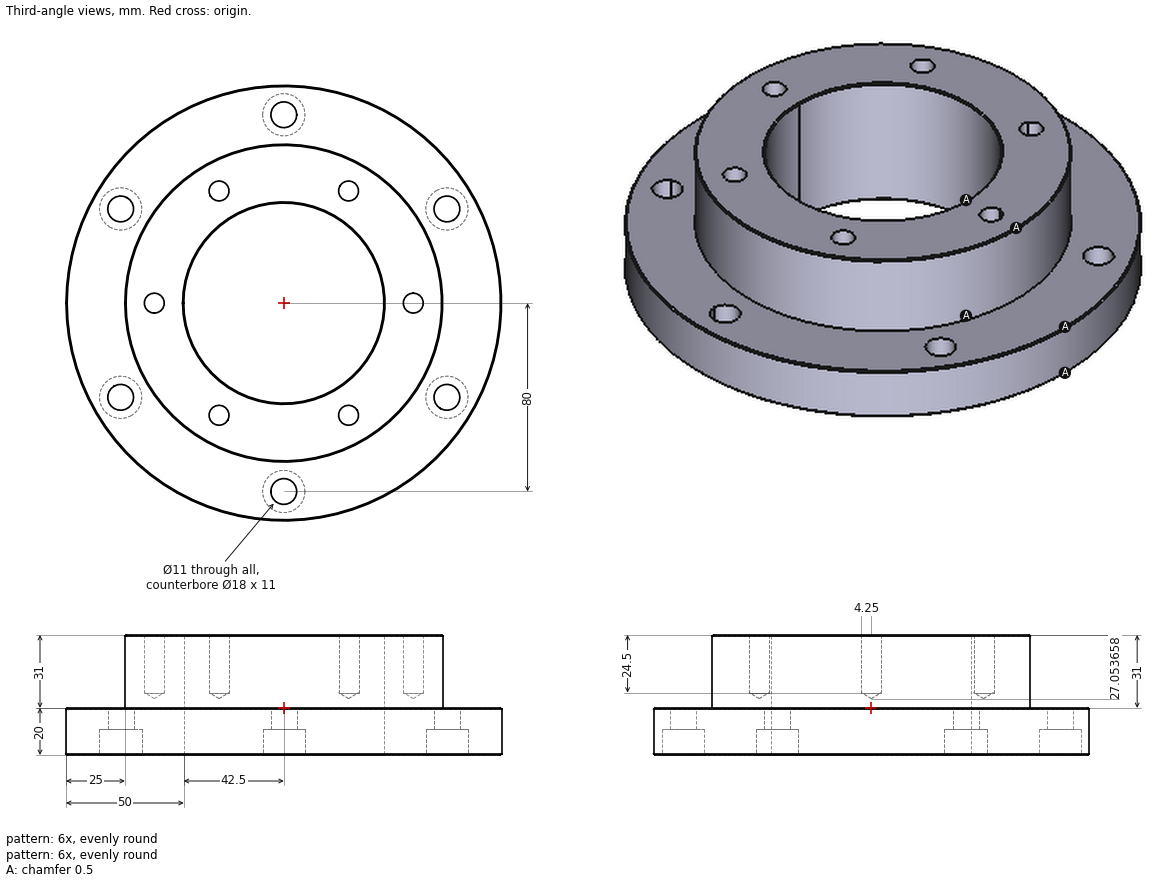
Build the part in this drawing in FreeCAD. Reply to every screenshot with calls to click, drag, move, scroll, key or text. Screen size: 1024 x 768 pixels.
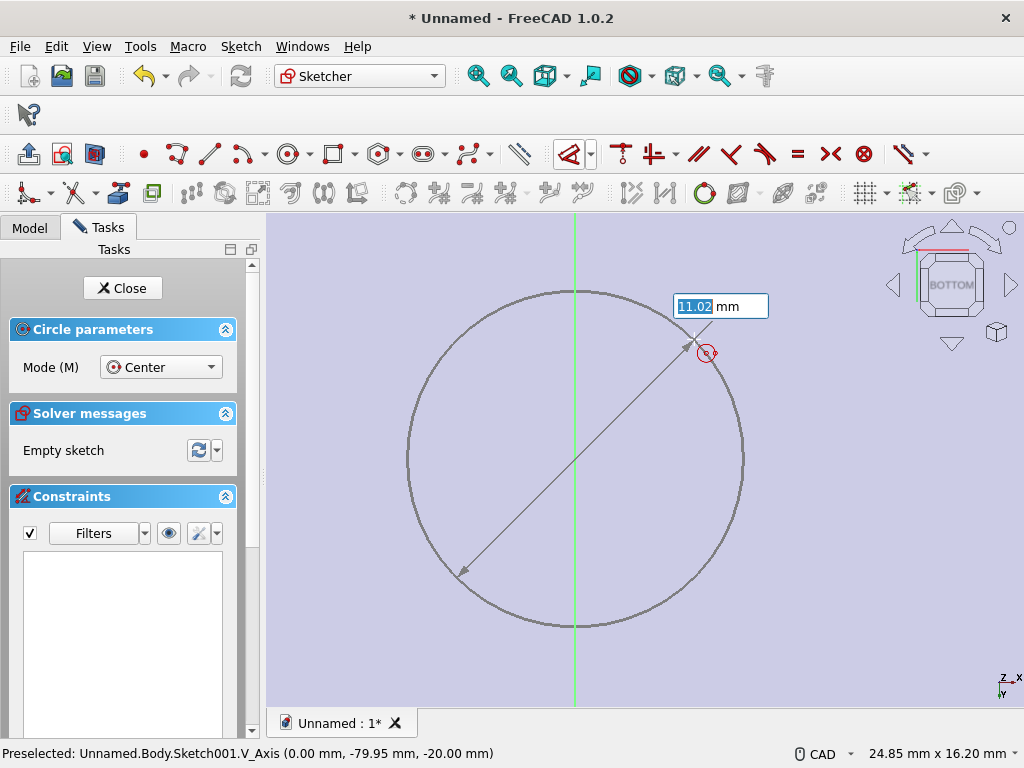
text(11)
key(Return)
key(Escape)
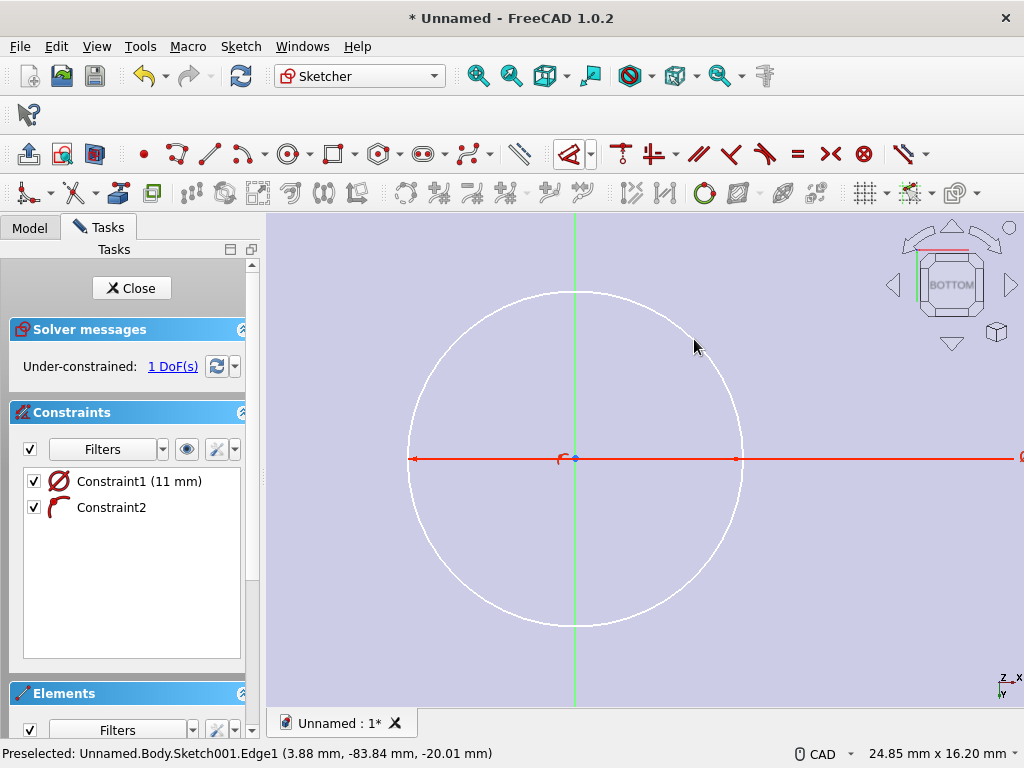
click(575, 459)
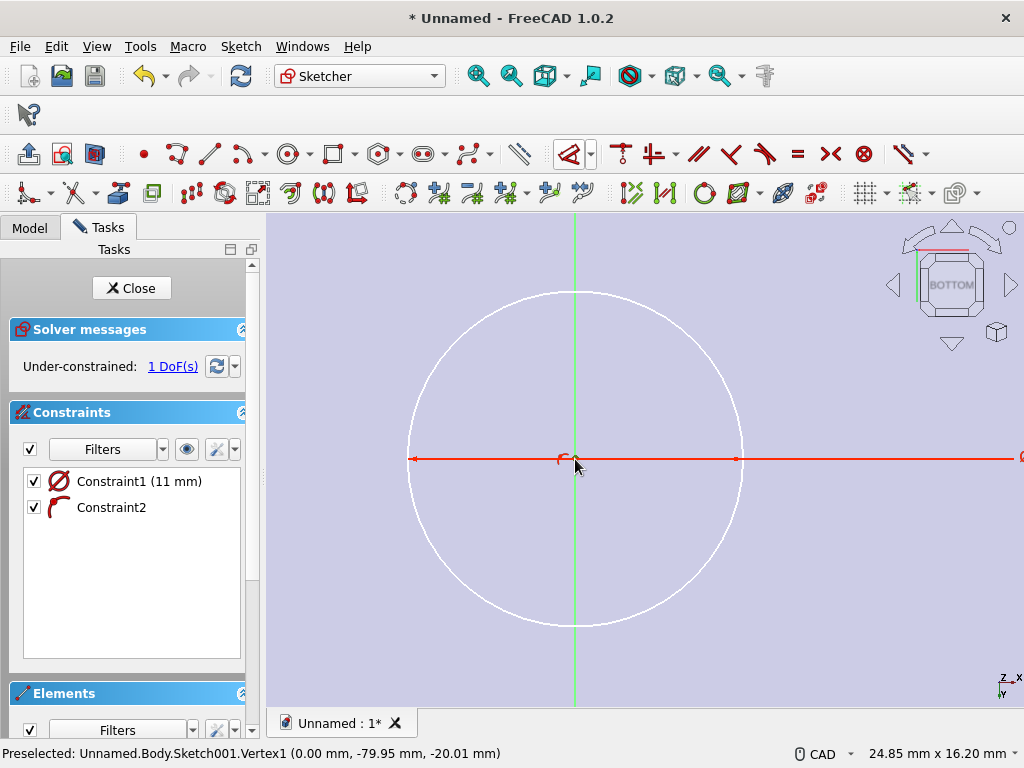
key(i)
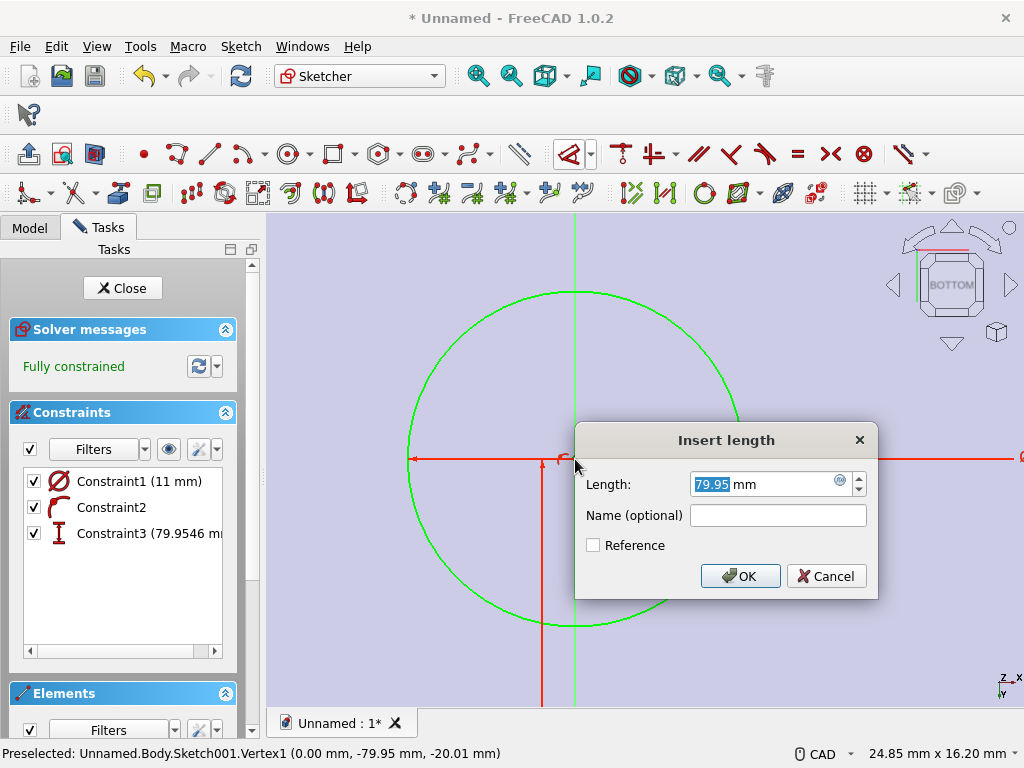
text(80)
key(Return)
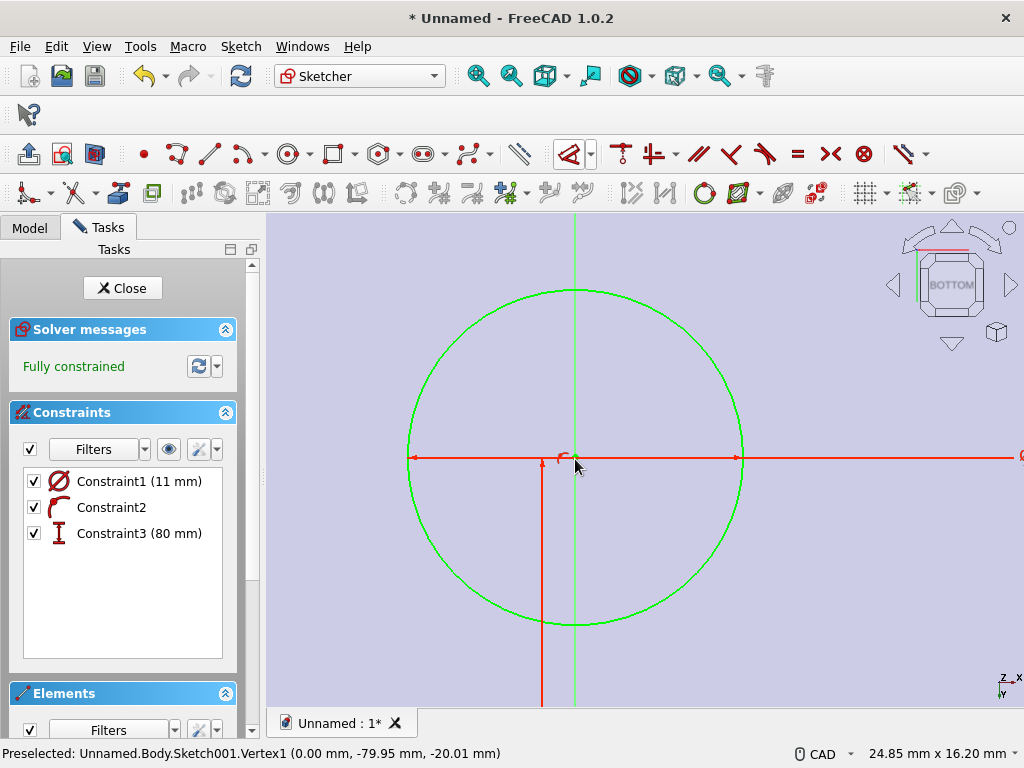
click(123, 288)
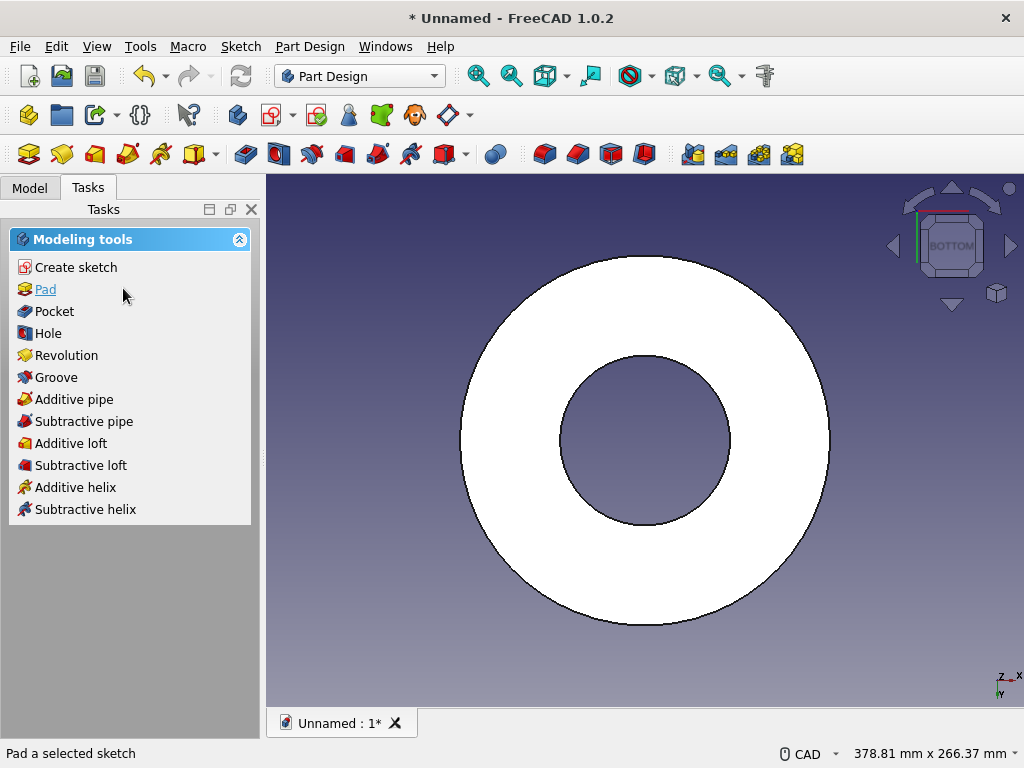
click(279, 154)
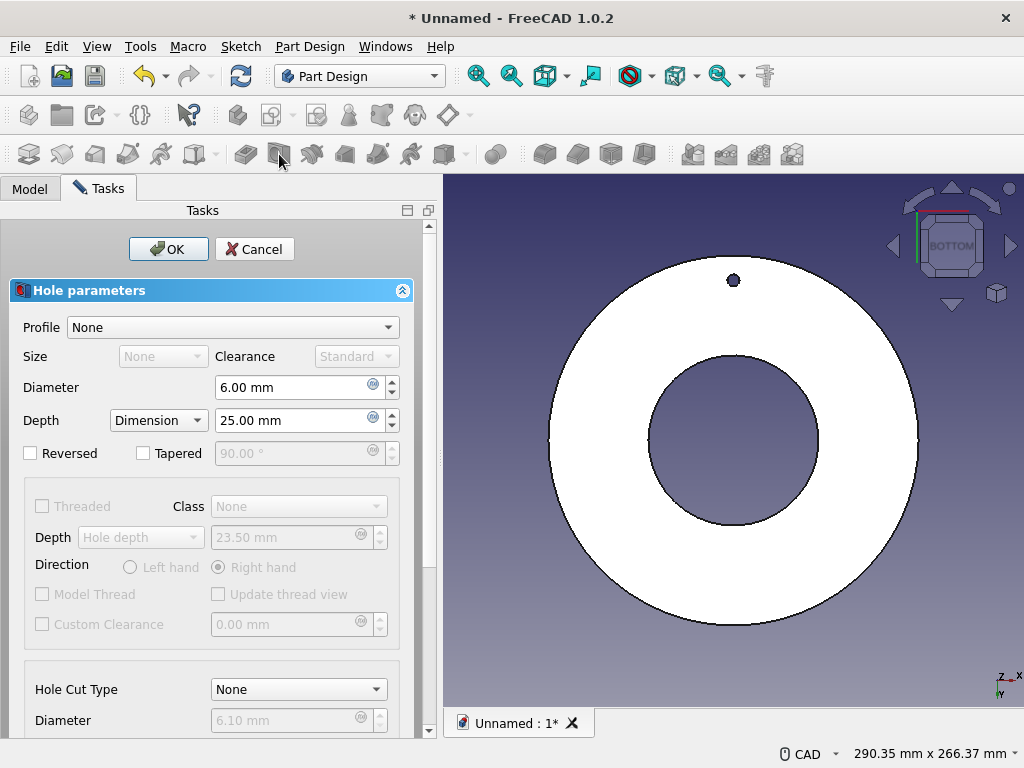
triple_click(300, 388)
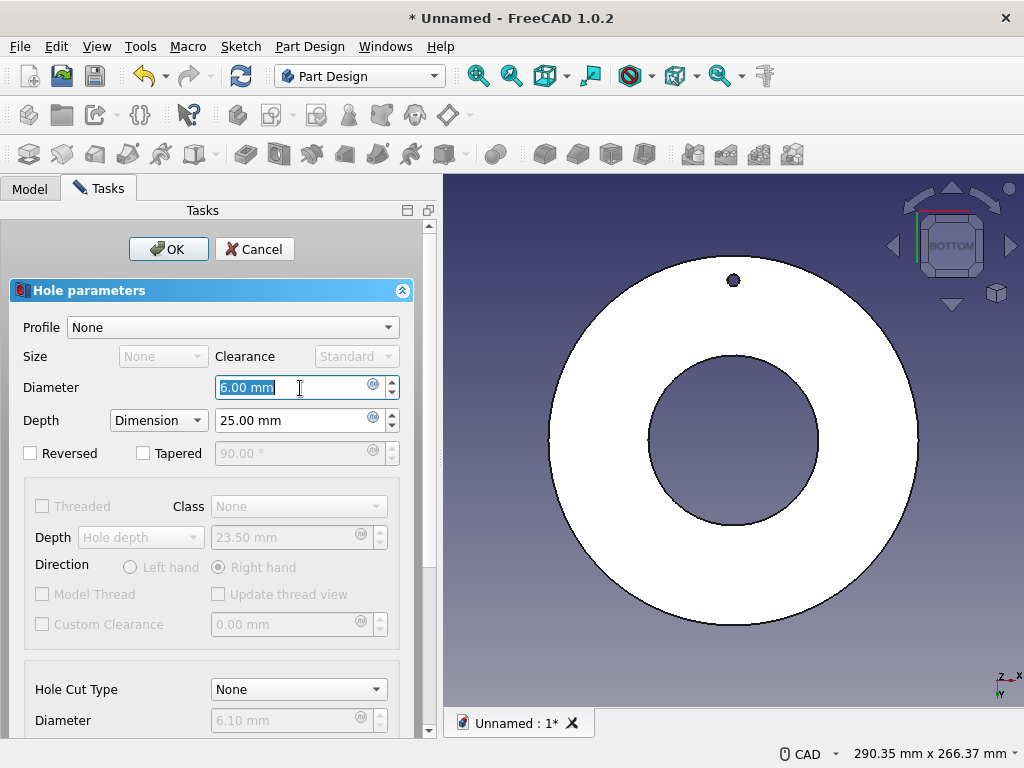
text(11)
key(Tab)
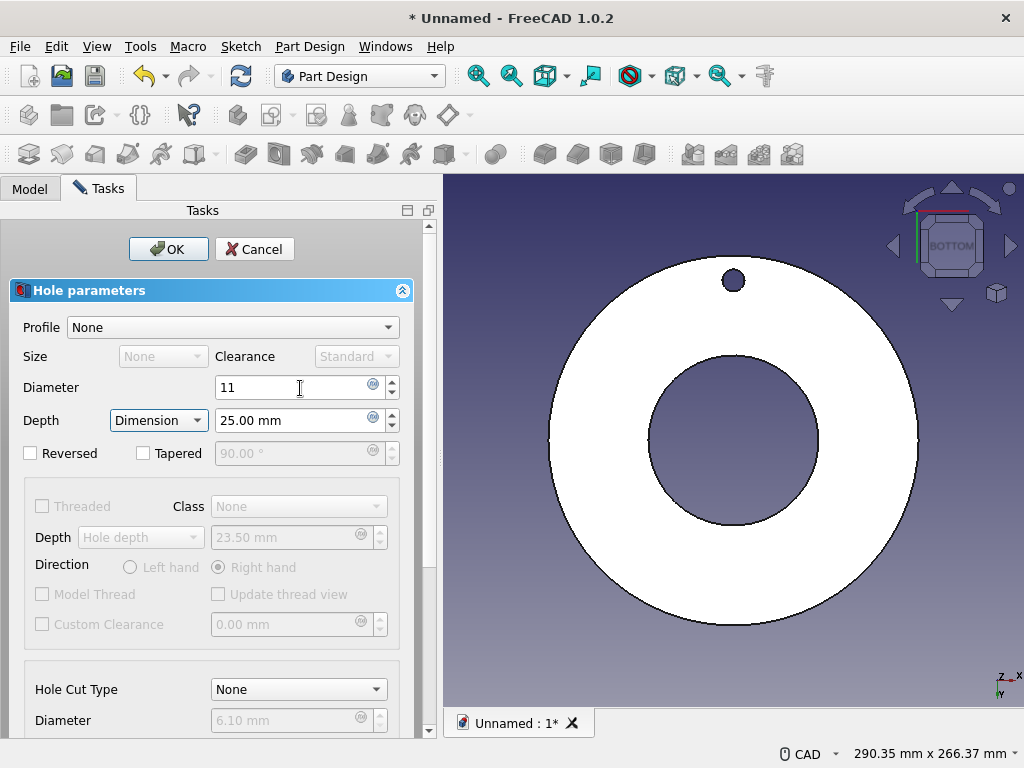
click(160, 420)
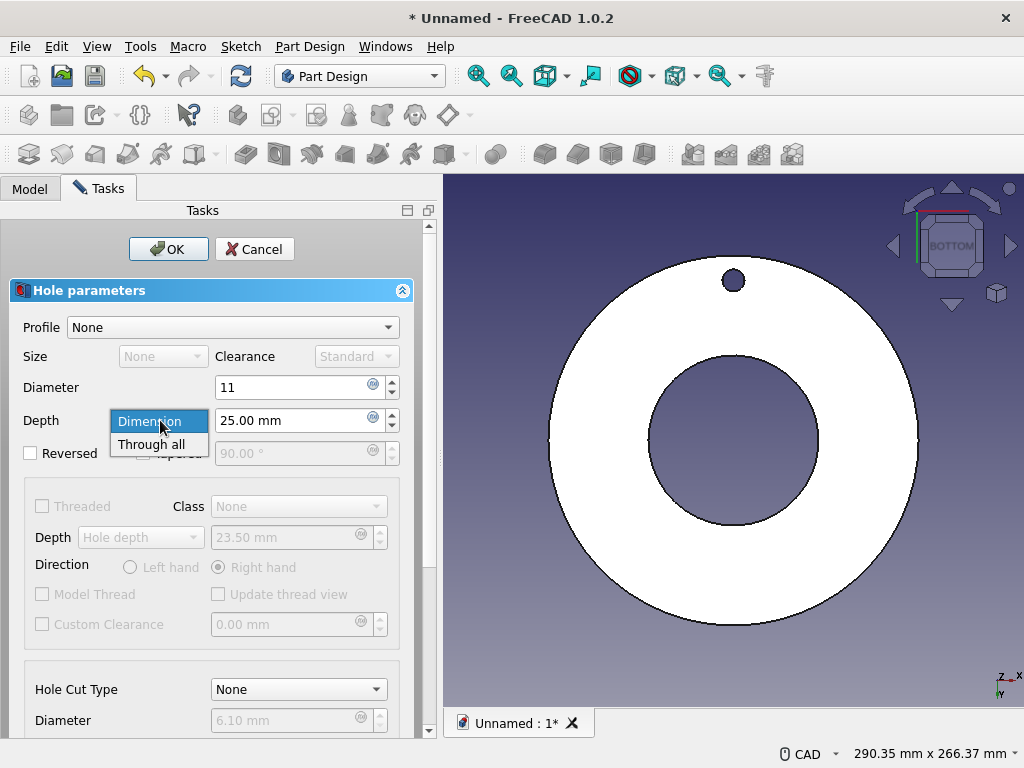
click(158, 444)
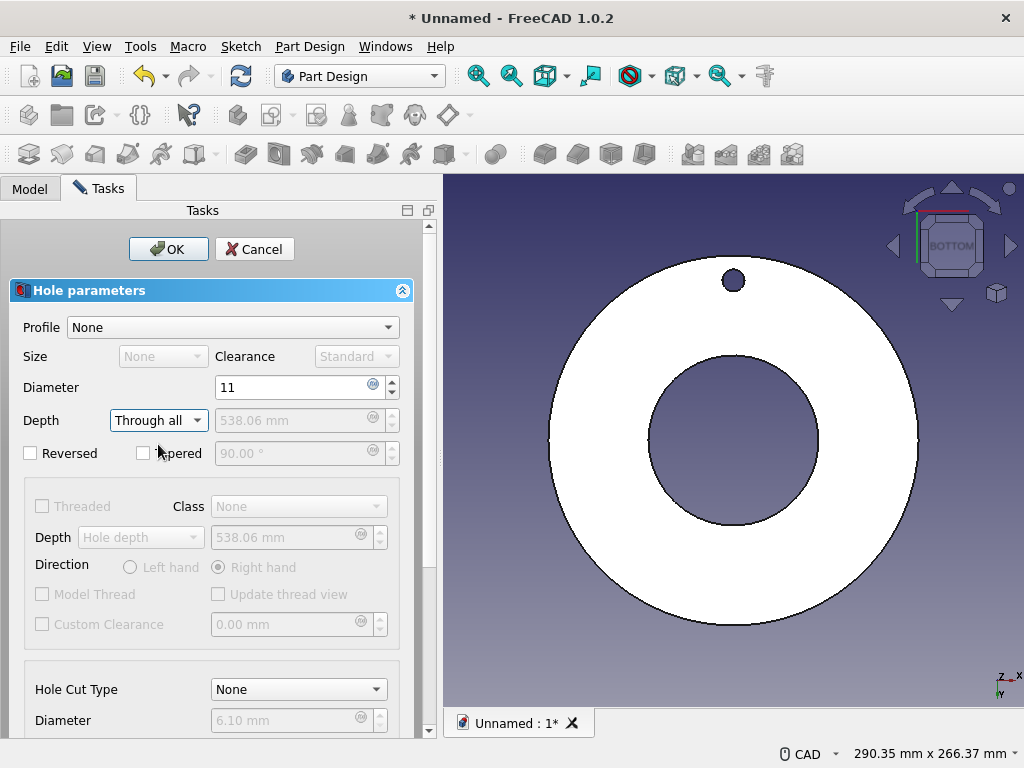
click(300, 690)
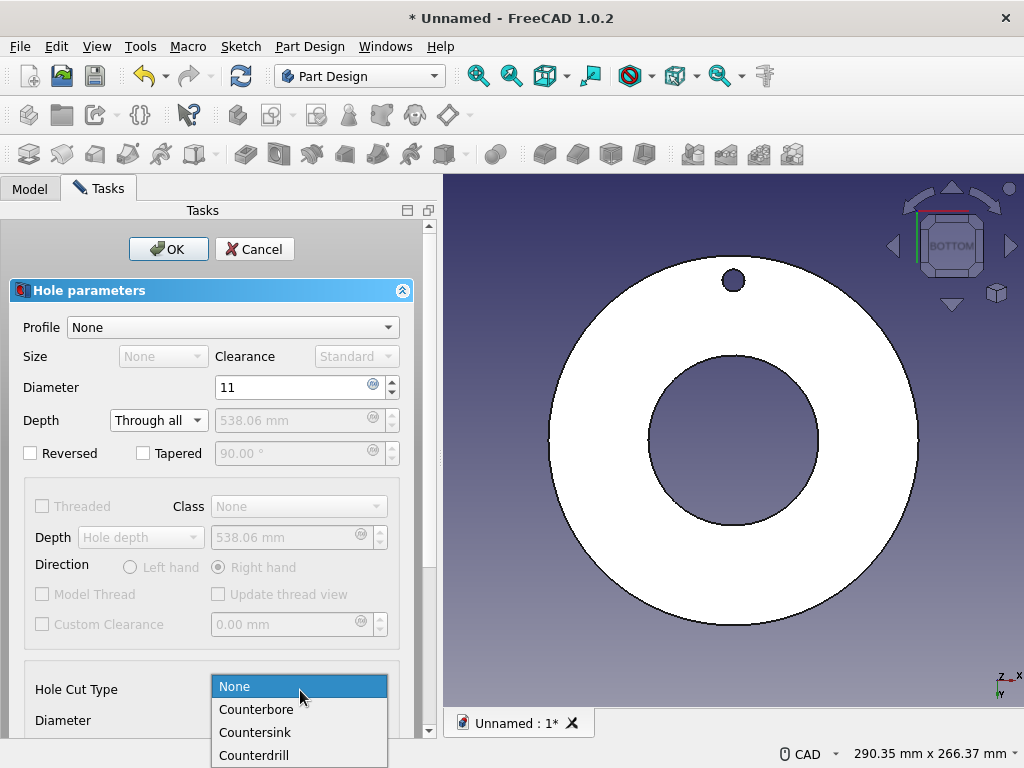
click(298, 710)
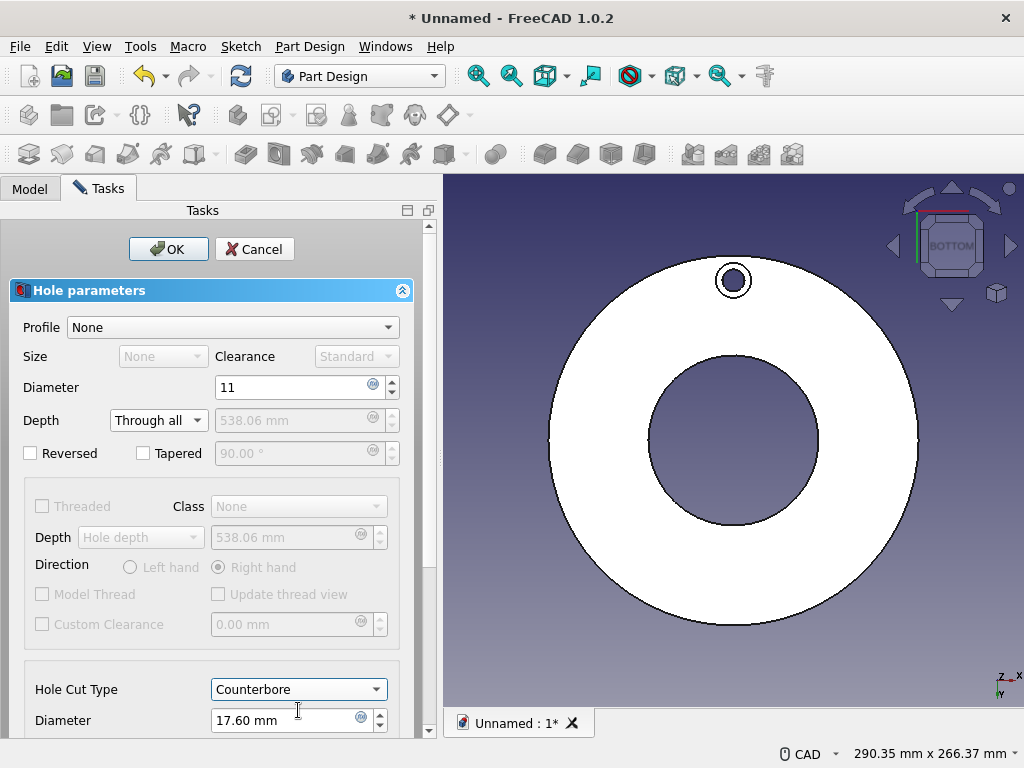
triple_click(292, 720)